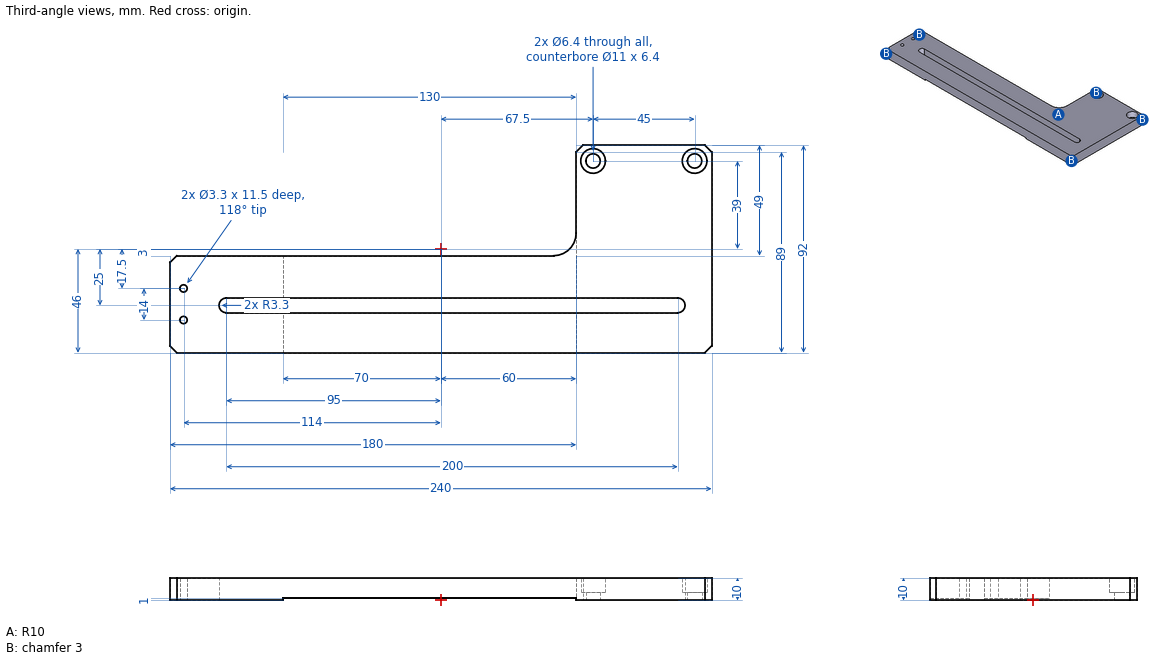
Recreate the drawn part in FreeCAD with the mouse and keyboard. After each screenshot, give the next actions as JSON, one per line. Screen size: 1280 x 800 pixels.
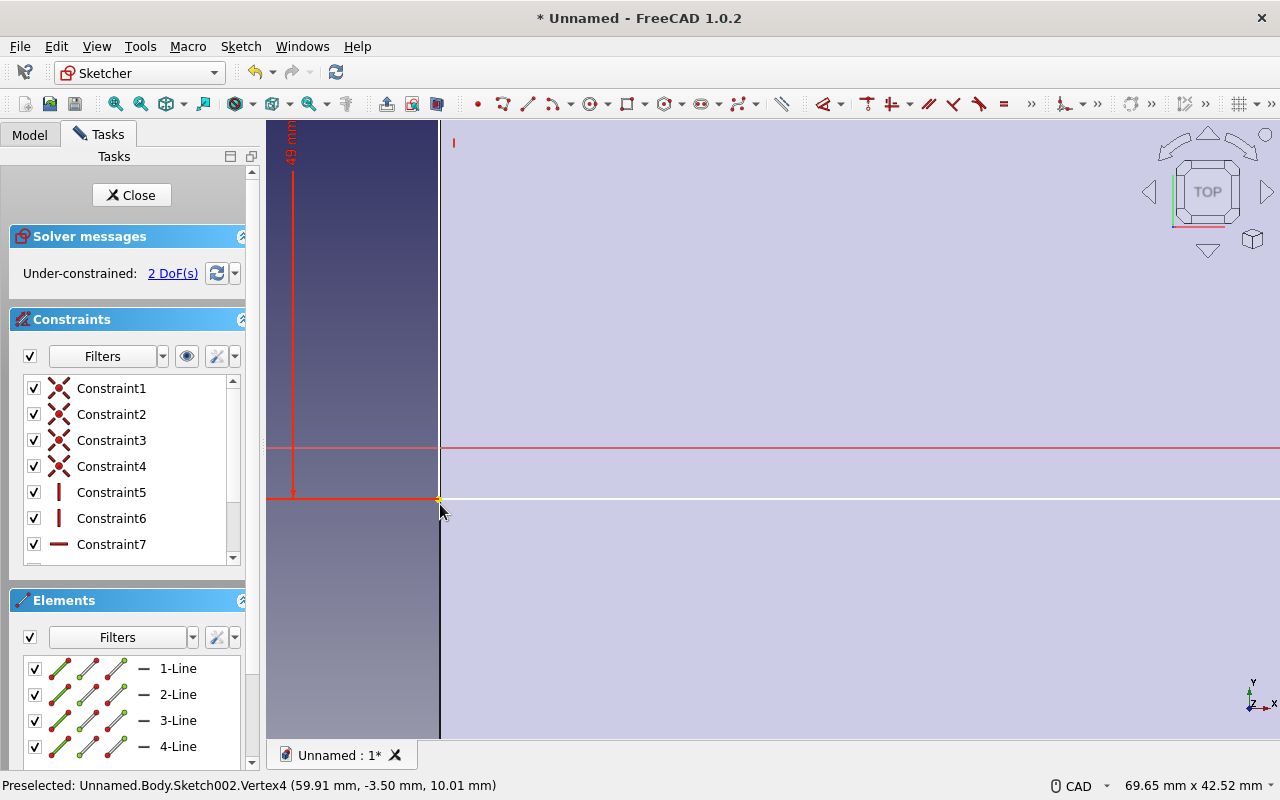
{"action": "left_click", "coordinate": [439, 499]}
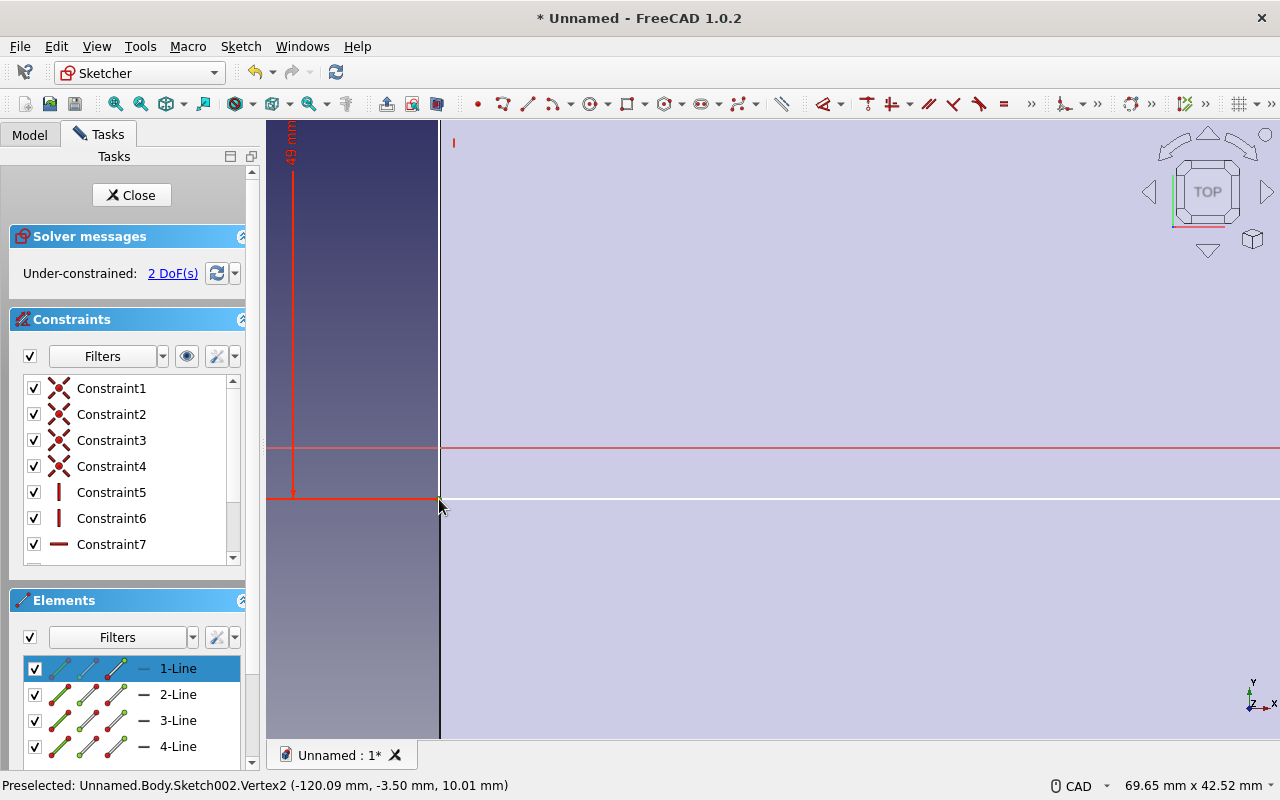
{"action": "key", "text": "i"}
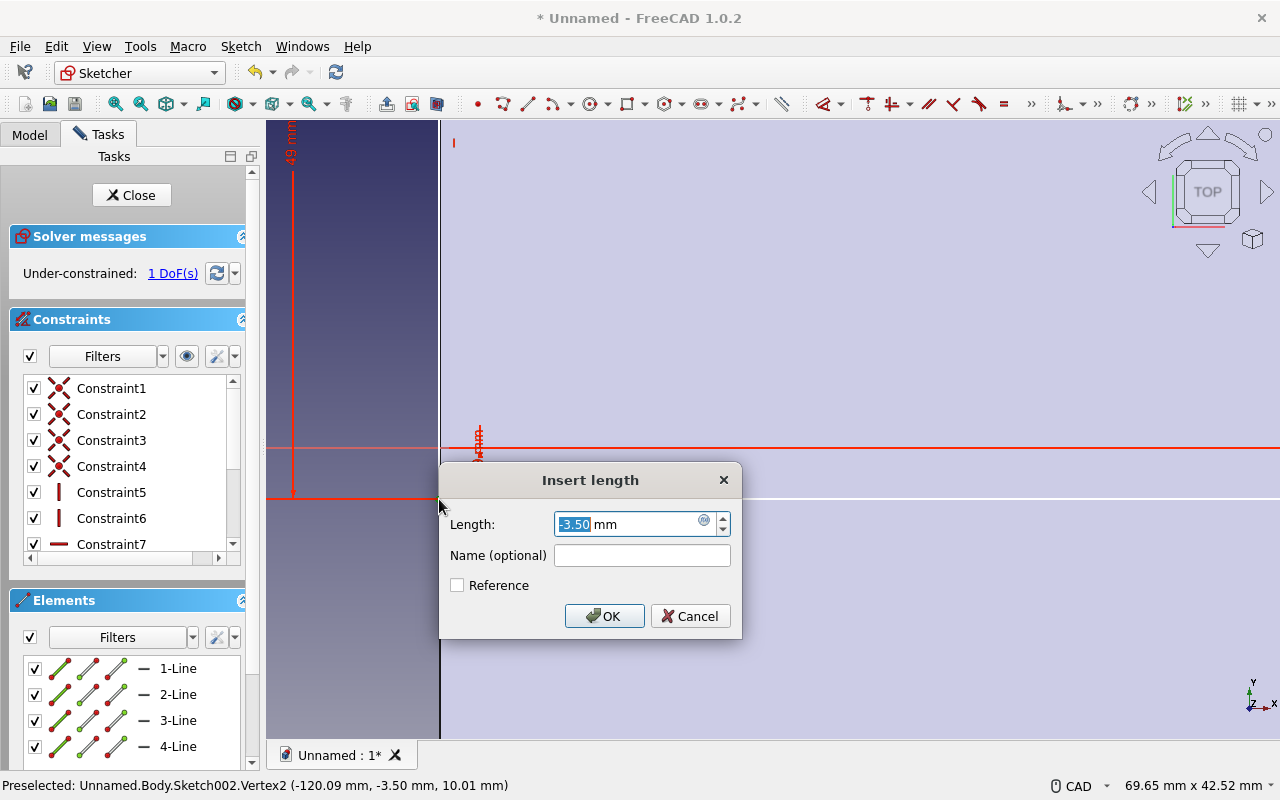
{"action": "type", "text": "-3"}
{"action": "key", "text": "Return"}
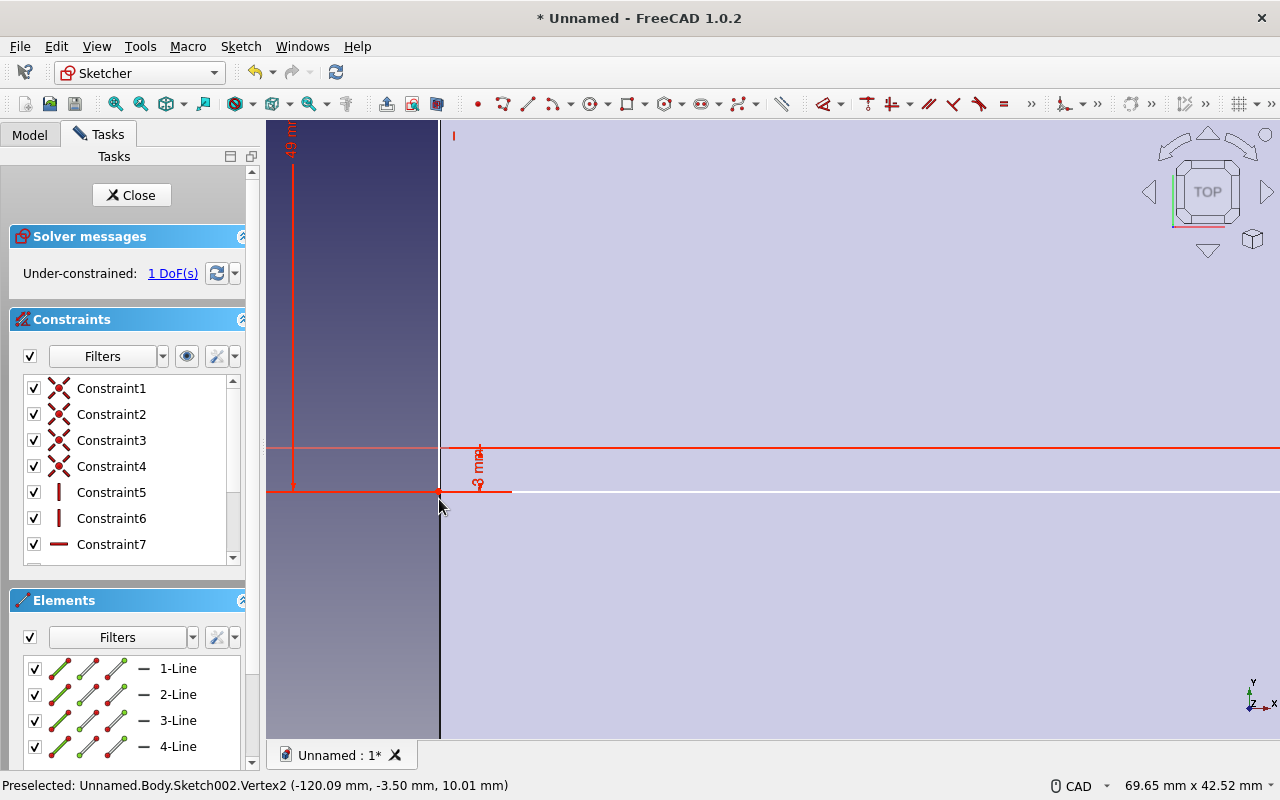
{"action": "scroll", "coordinate": [440, 504], "scroll_direction": "down", "scroll_amount": 8}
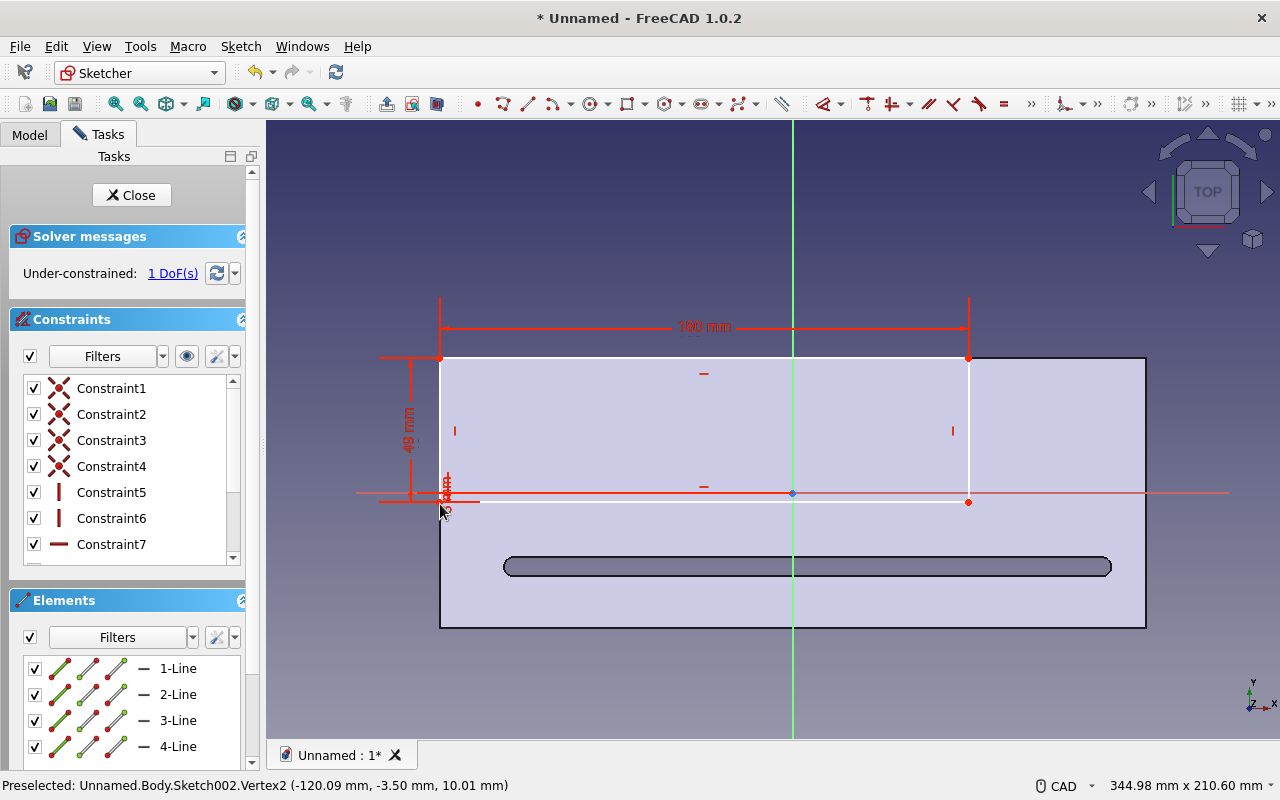
{"action": "left_click", "coordinate": [969, 502]}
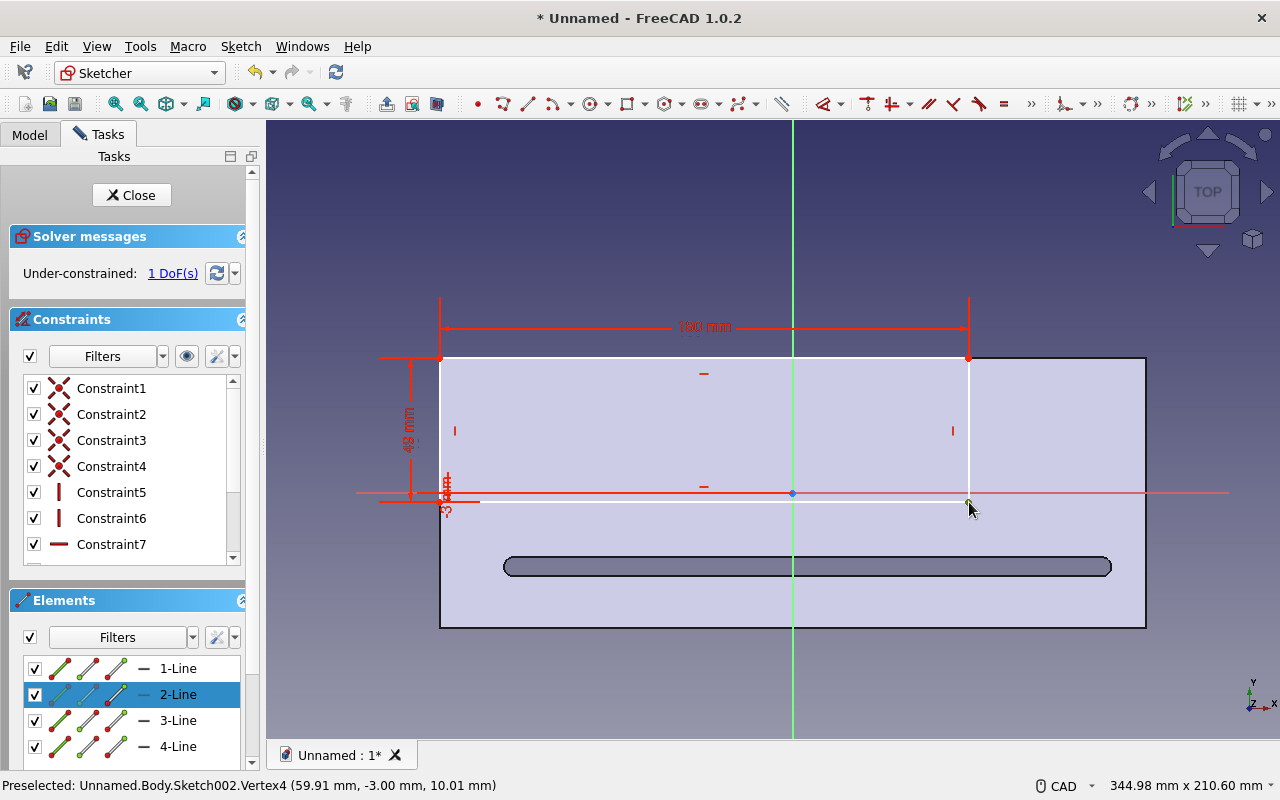
{"action": "key", "text": "l"}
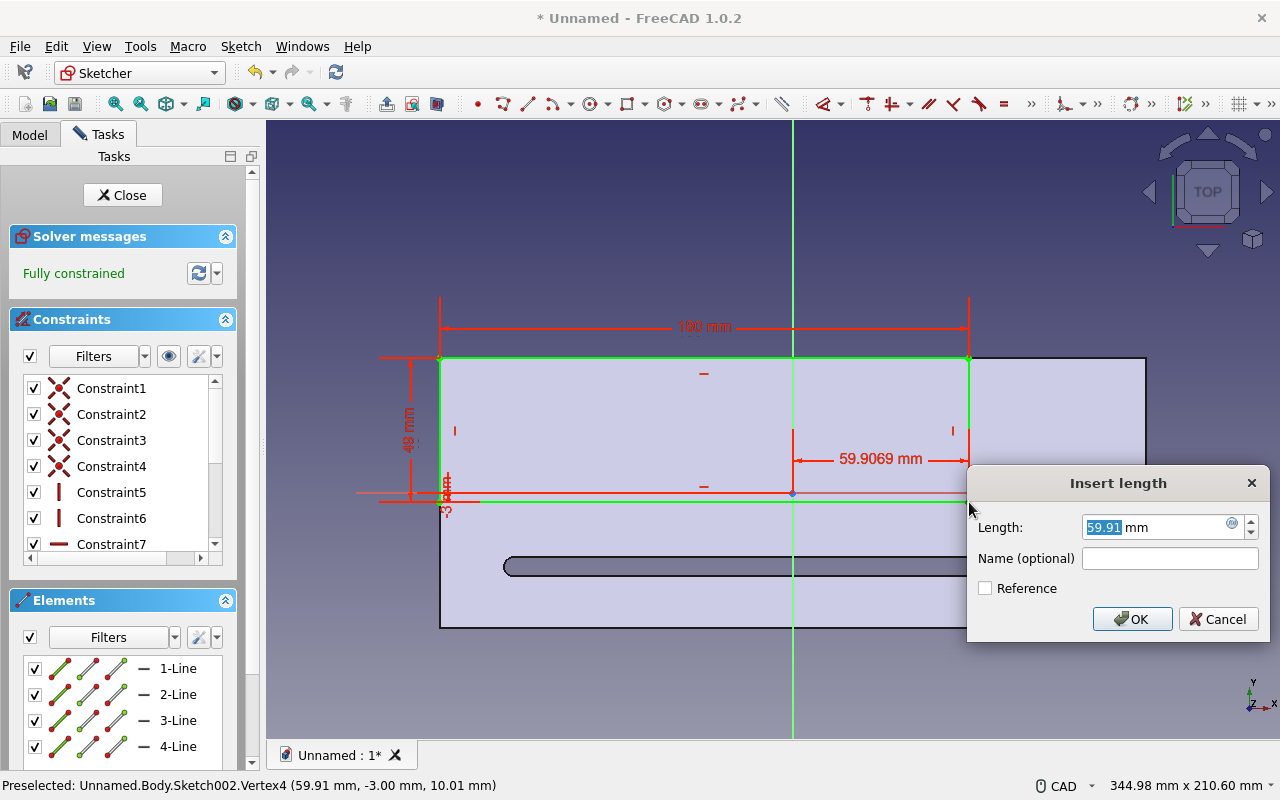
{"action": "type", "text": "60"}
{"action": "key", "text": "Return"}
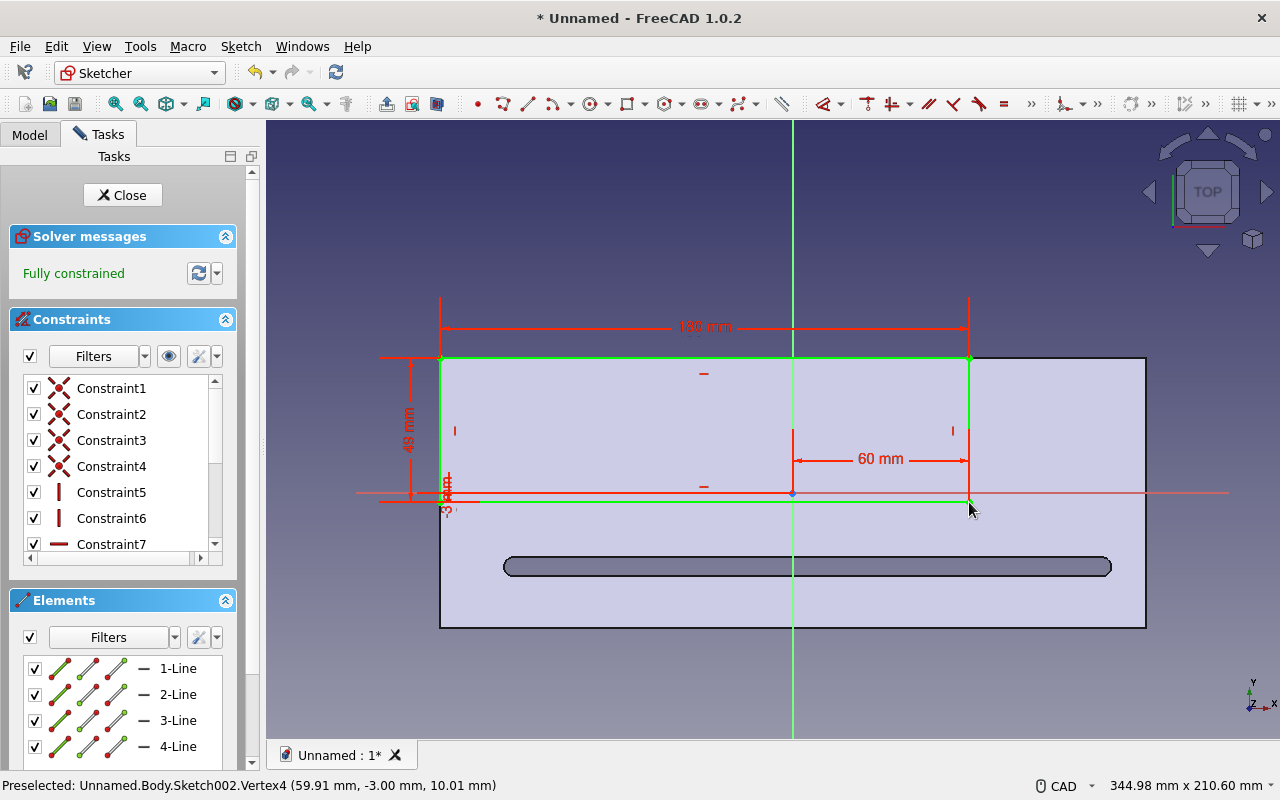
{"action": "left_click", "coordinate": [123, 195]}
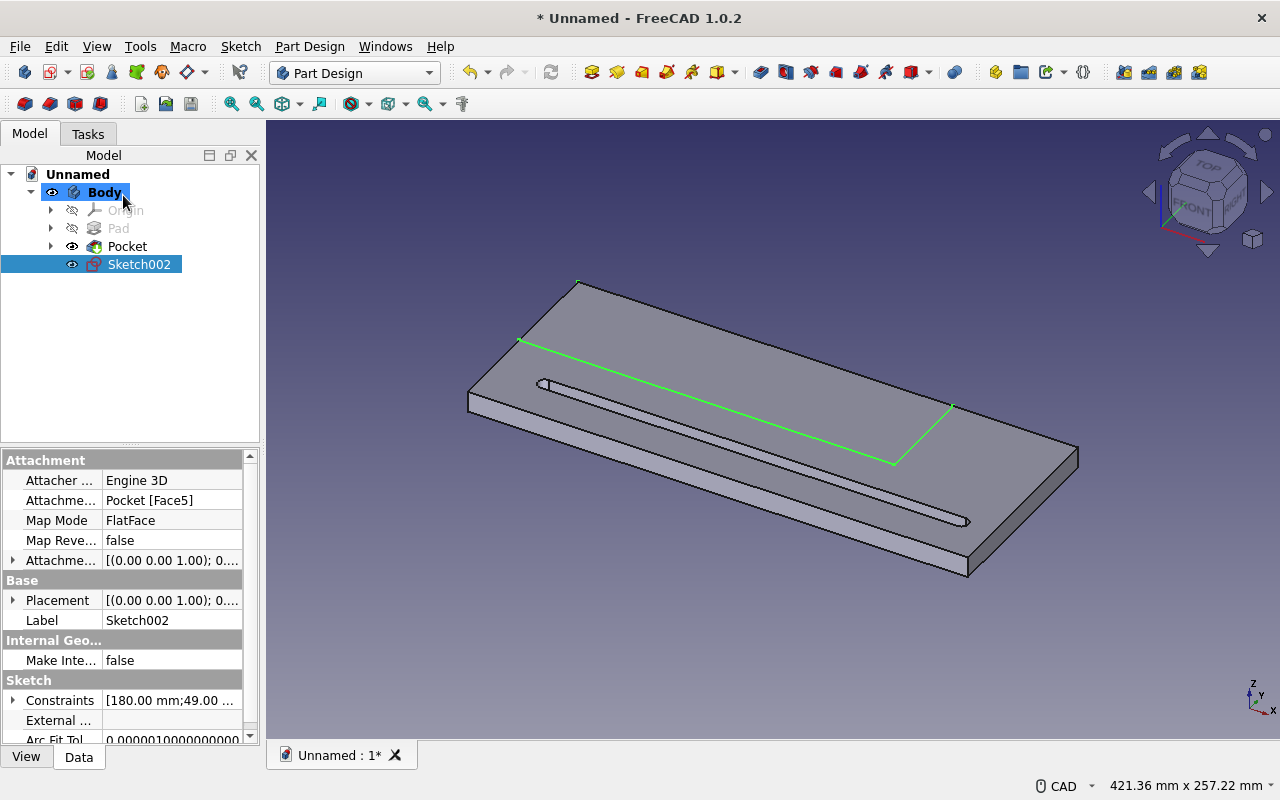
{"action": "left_click", "coordinate": [761, 72]}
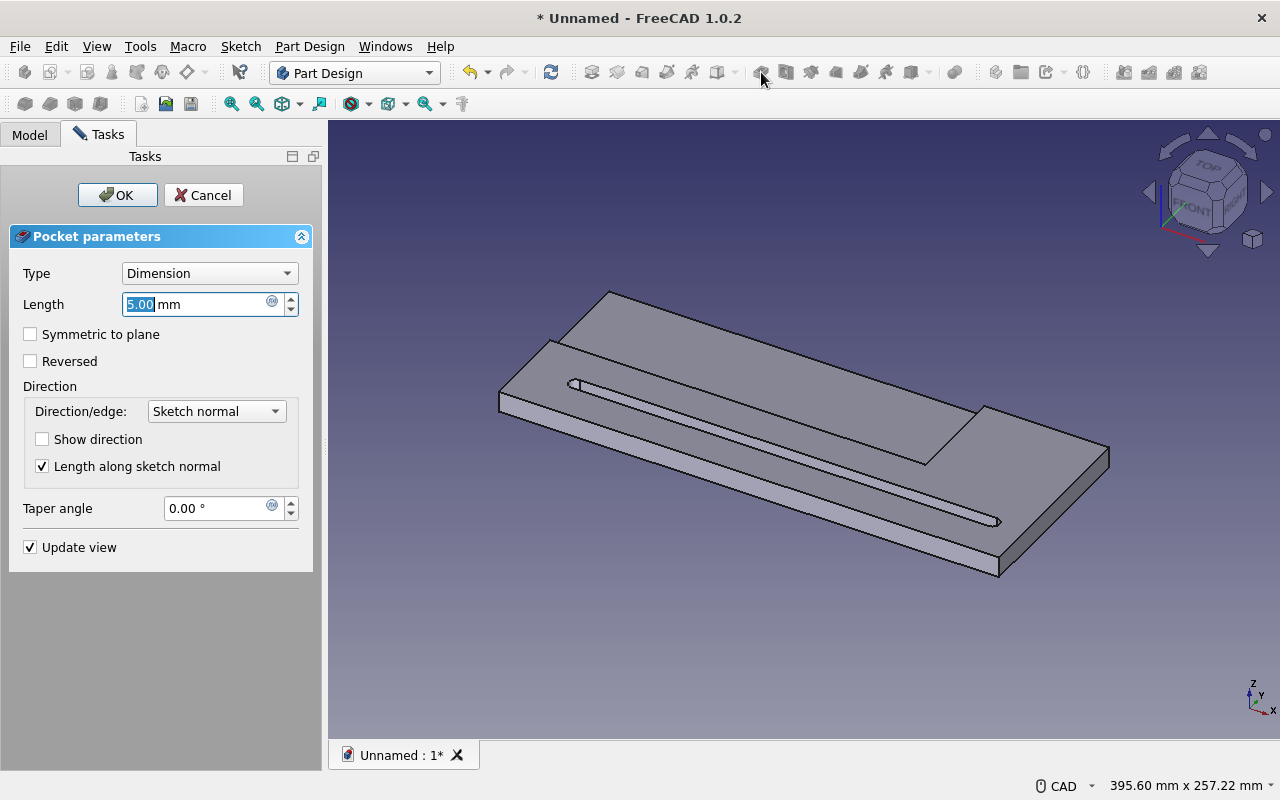
{"action": "type", "text": "10"}
{"action": "key", "text": "Tab"}